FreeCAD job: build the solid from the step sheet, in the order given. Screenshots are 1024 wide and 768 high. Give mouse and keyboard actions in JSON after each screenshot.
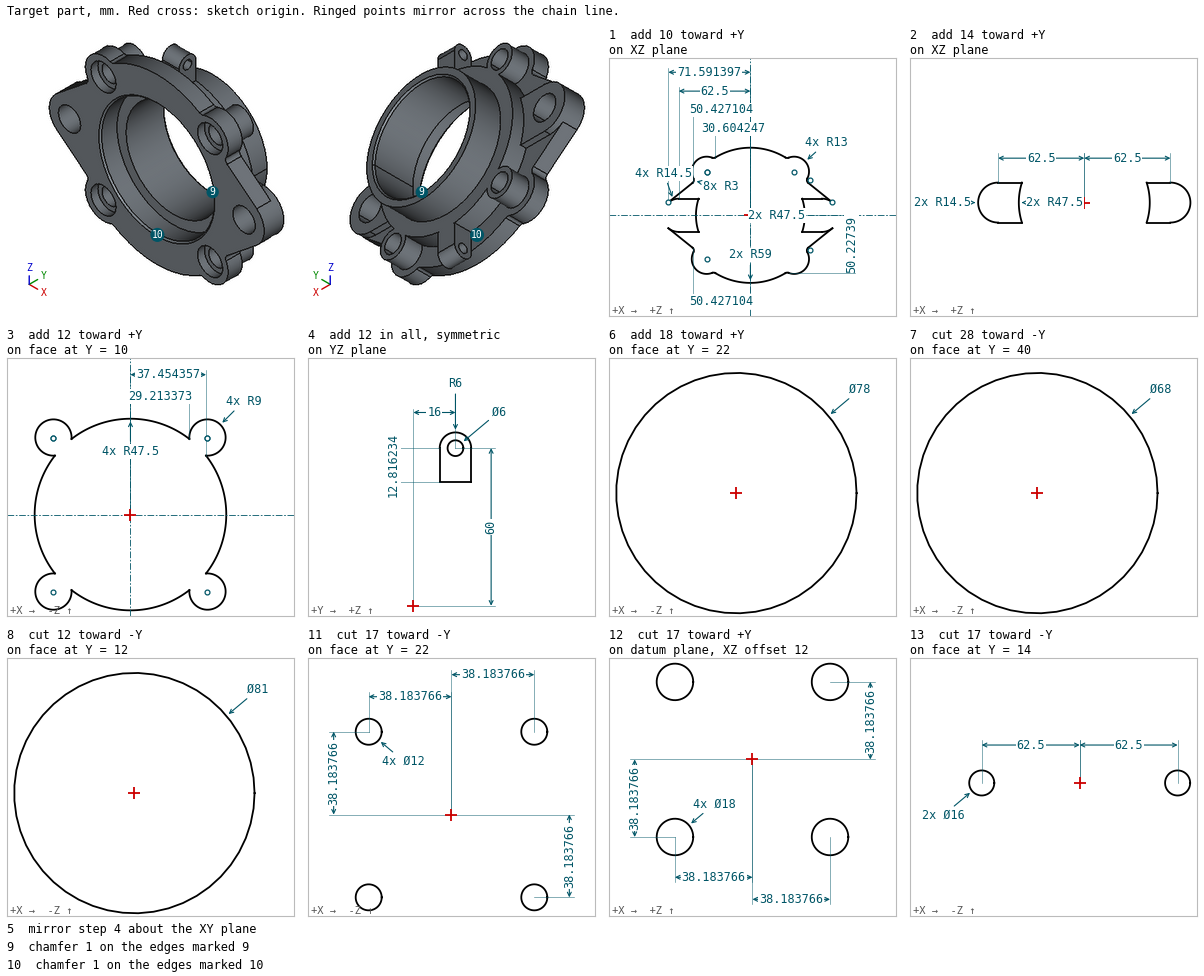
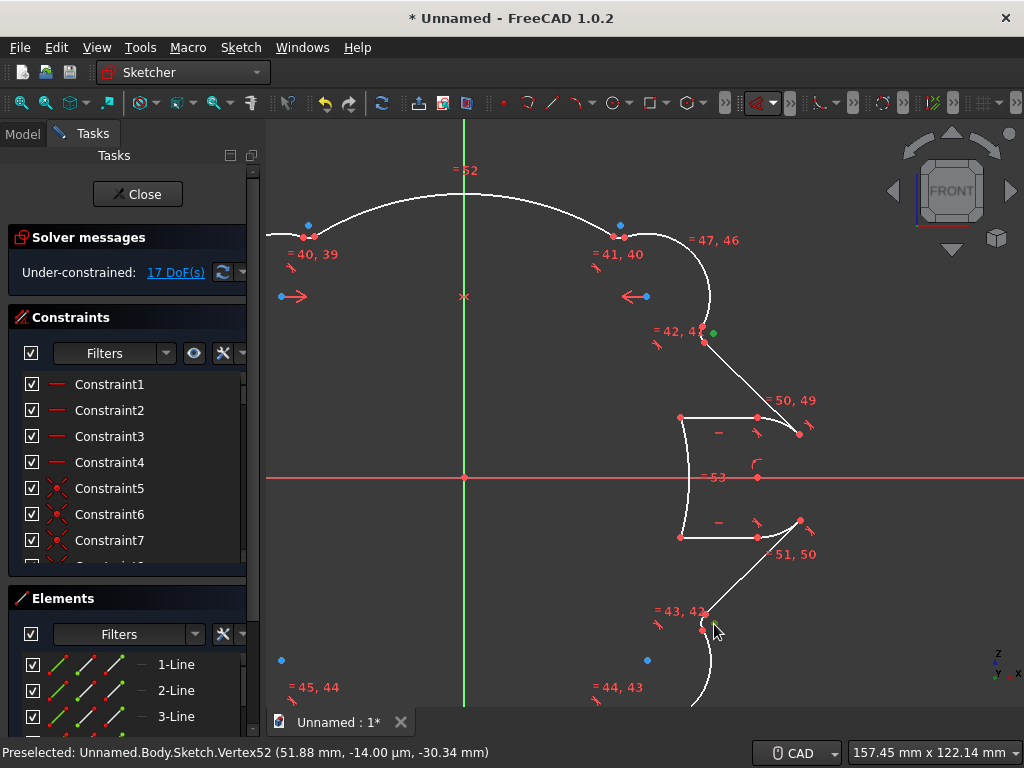
{"action": "left_click", "coordinate": [334, 478]}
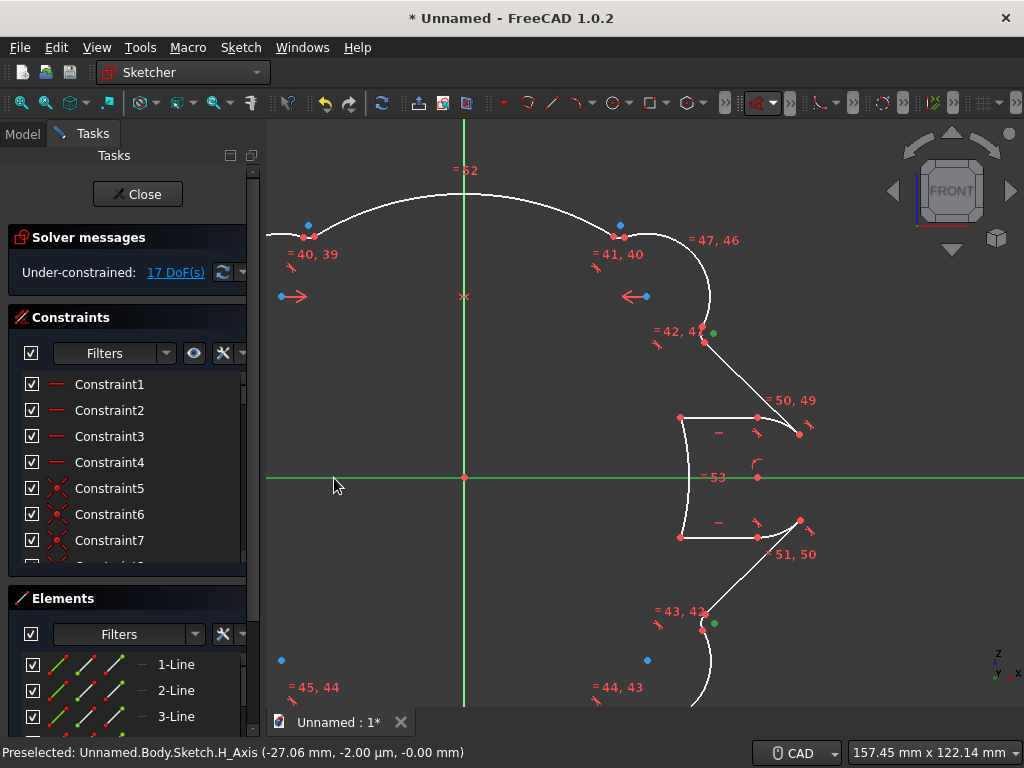
{"action": "key", "text": "s"}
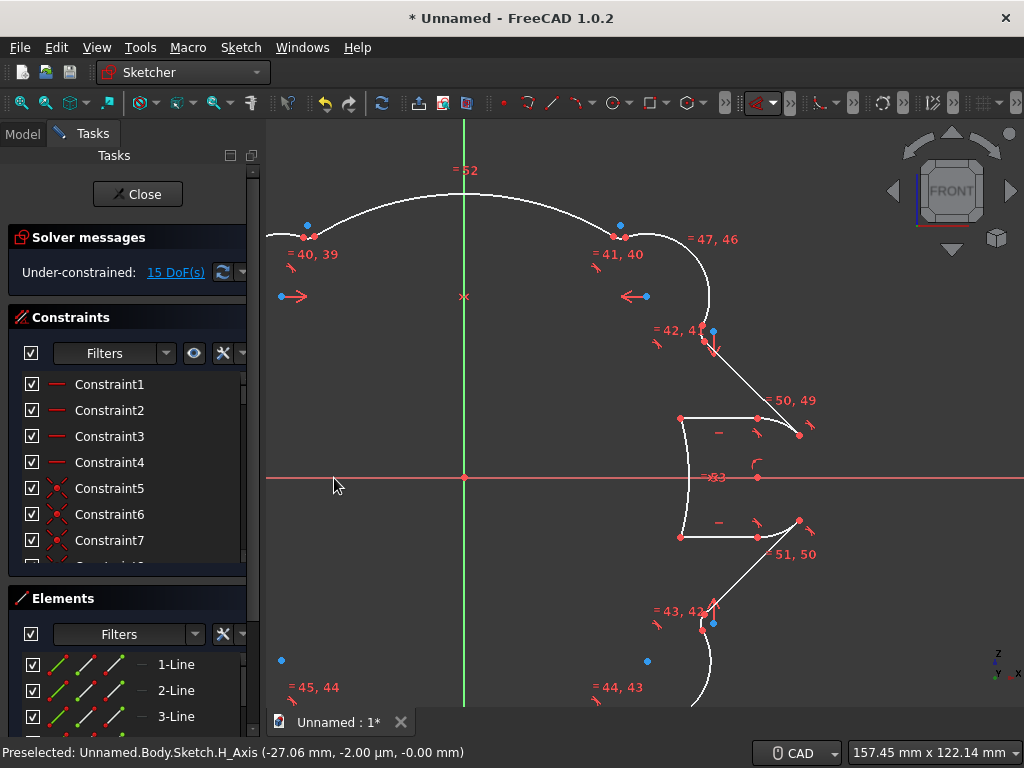
{"action": "scroll", "coordinate": [713, 334], "scroll_direction": "down", "scroll_amount": 3}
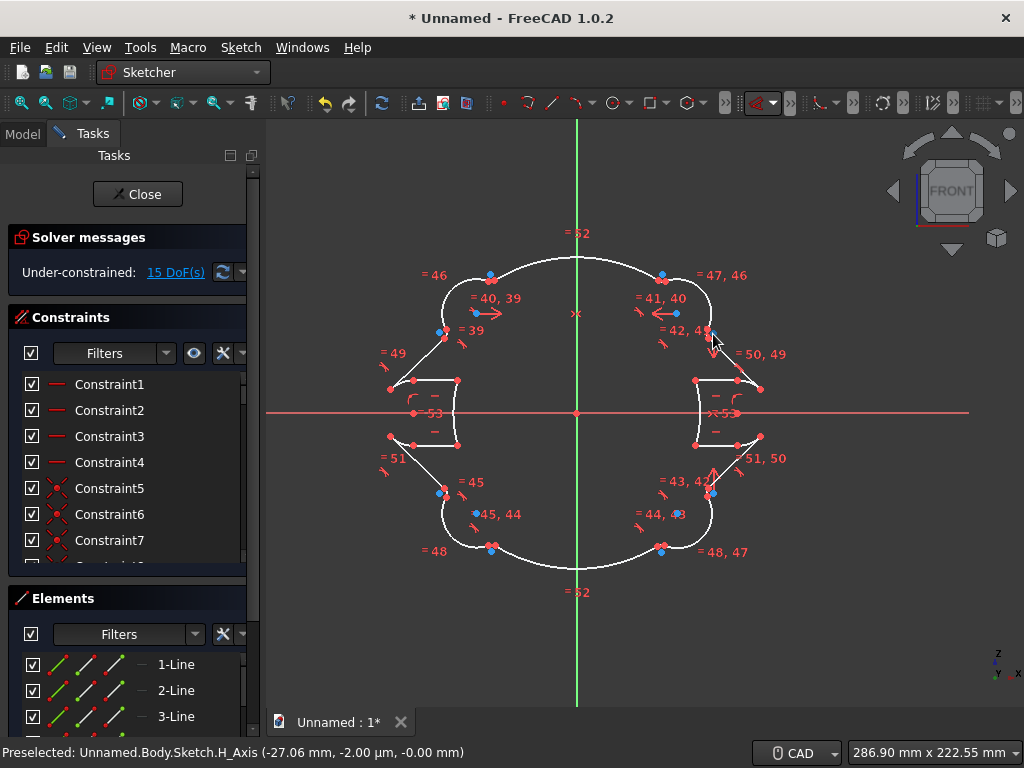
{"action": "left_click", "coordinate": [477, 314]}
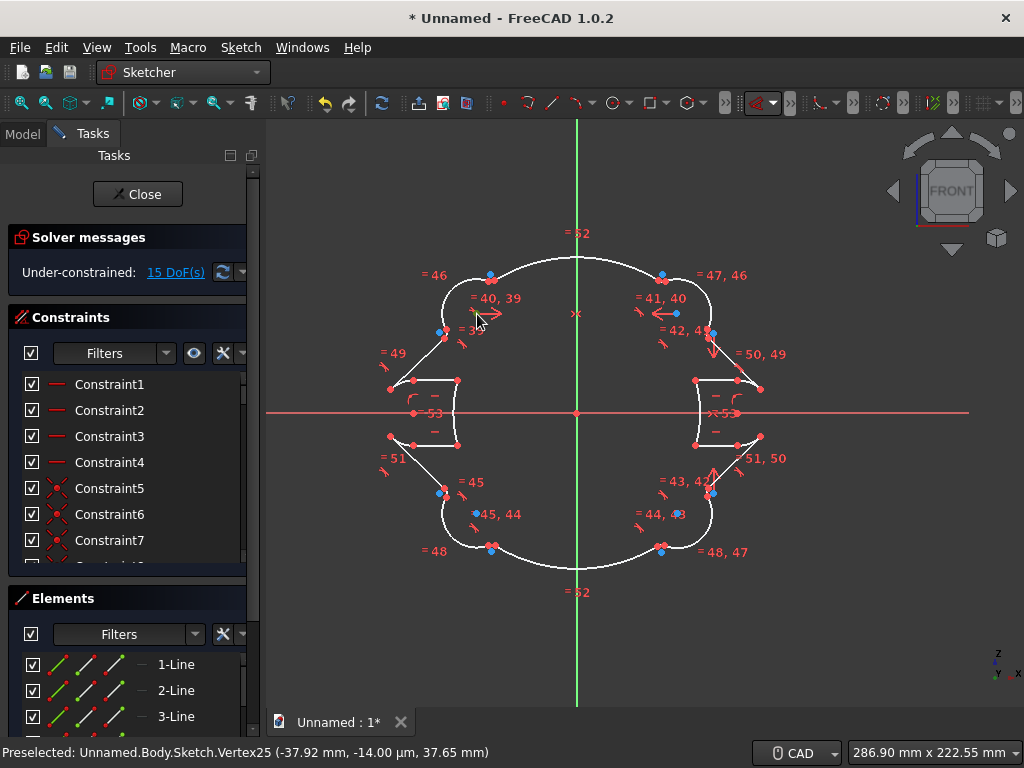
{"action": "left_click", "coordinate": [477, 513]}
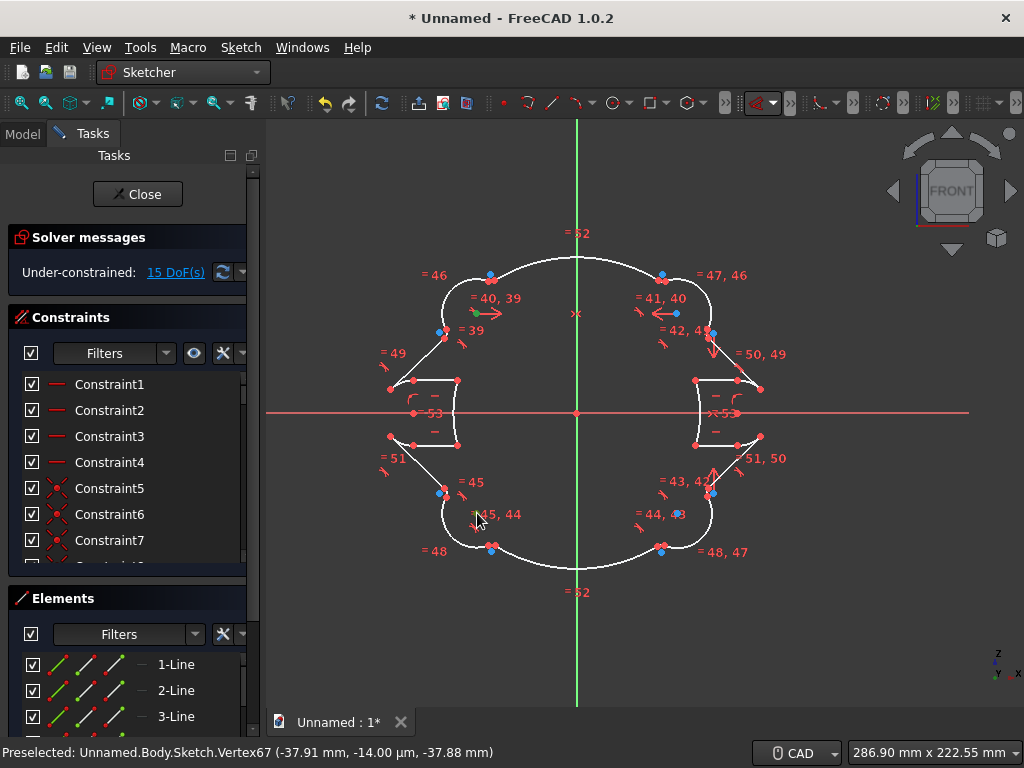
{"action": "left_click", "coordinate": [334, 413]}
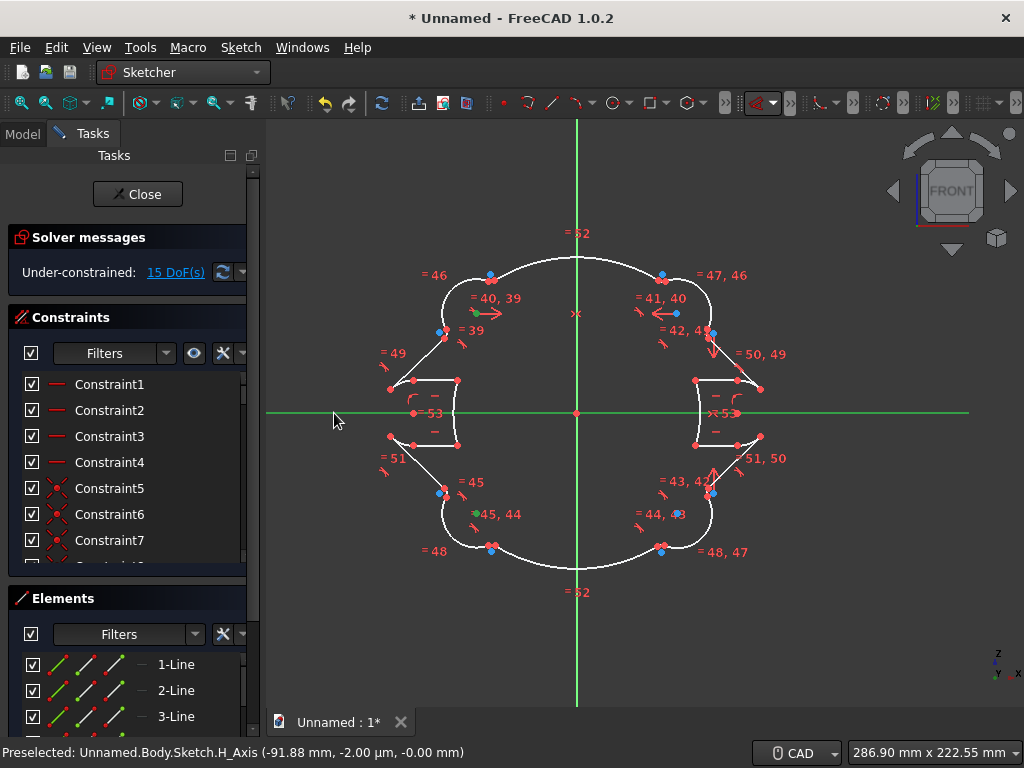
{"action": "key", "text": "s"}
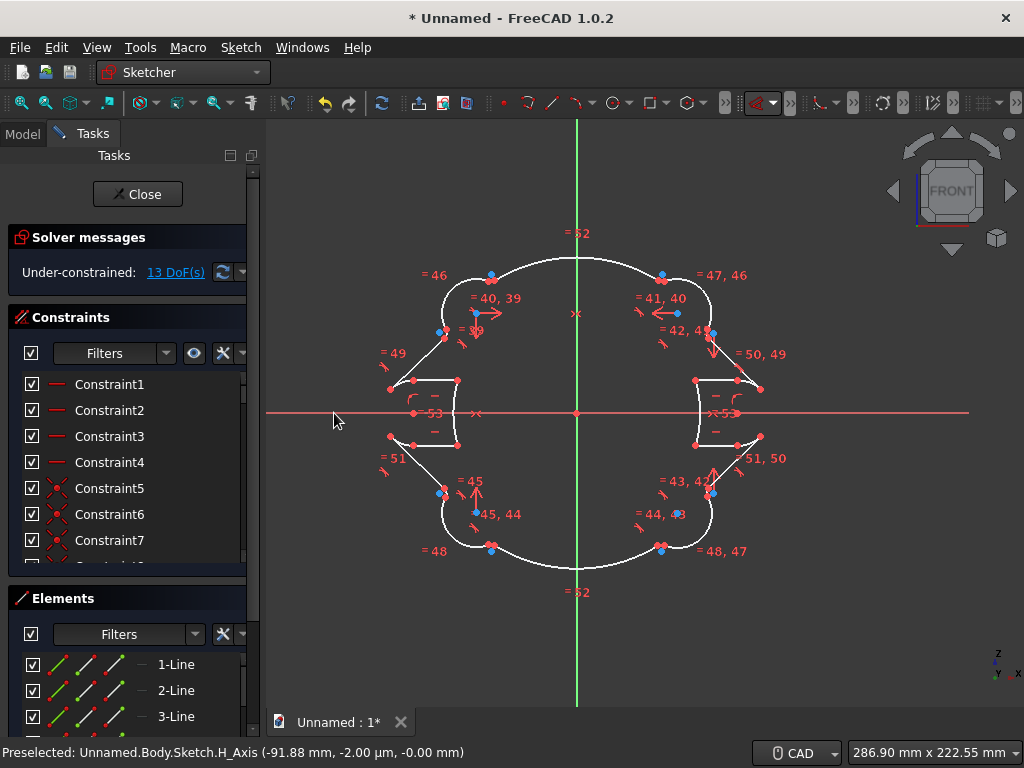
{"action": "left_click", "coordinate": [391, 389]}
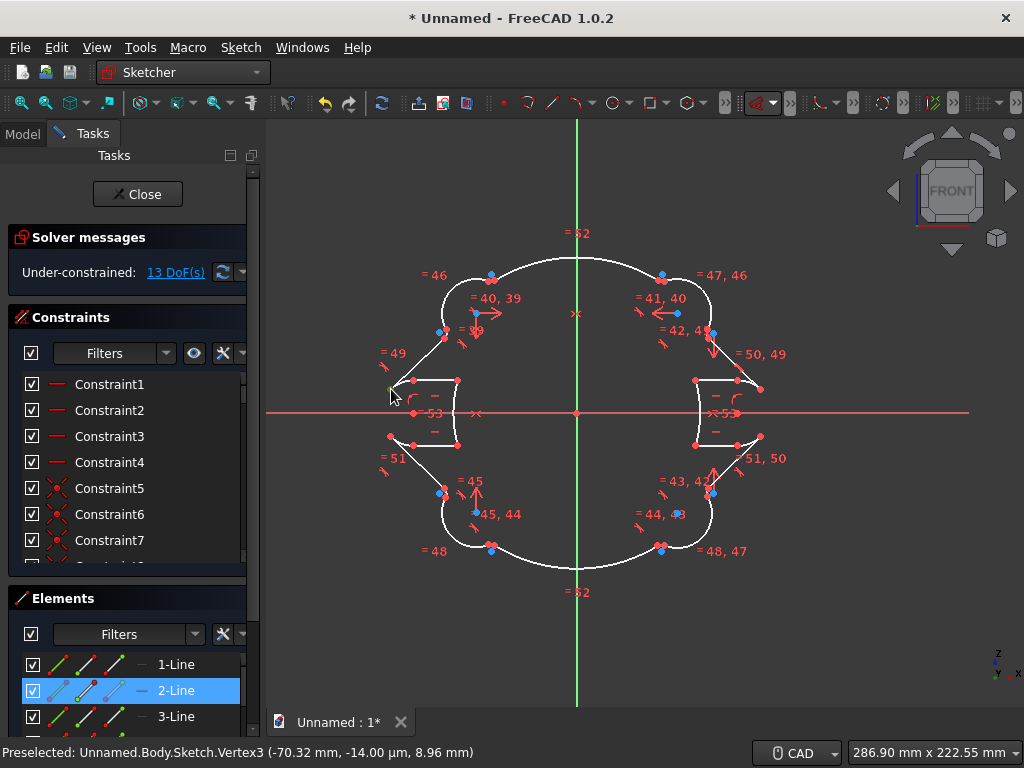
{"action": "left_click", "coordinate": [761, 390]}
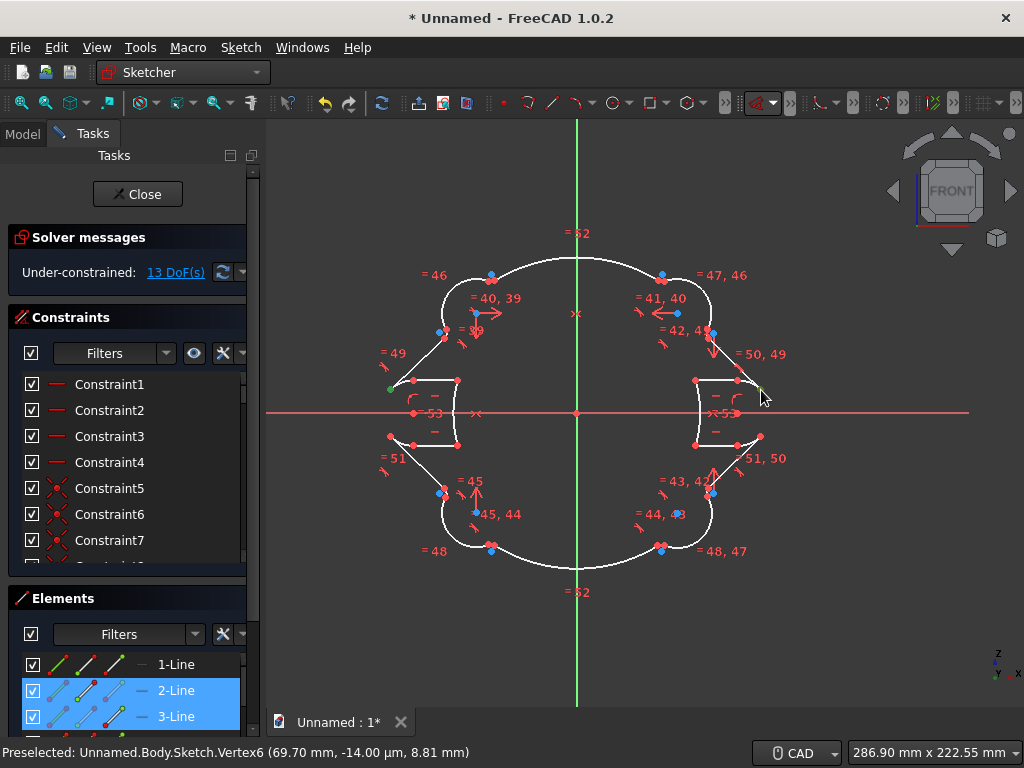
{"action": "left_click", "coordinate": [577, 641]}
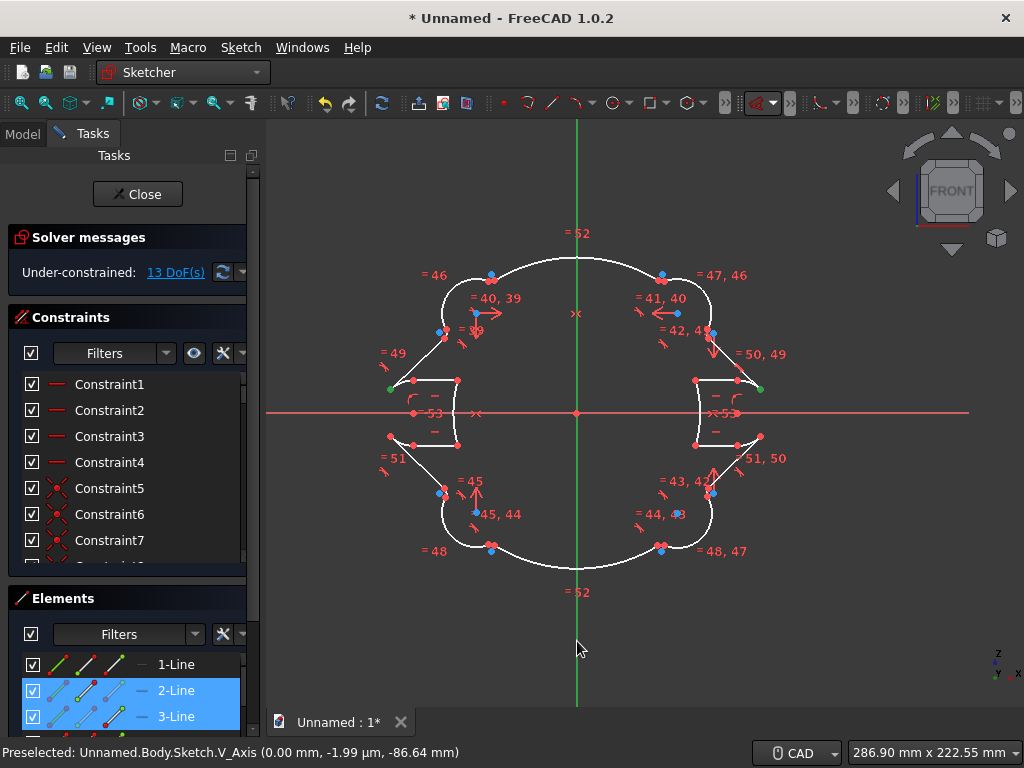
{"action": "key", "text": "s"}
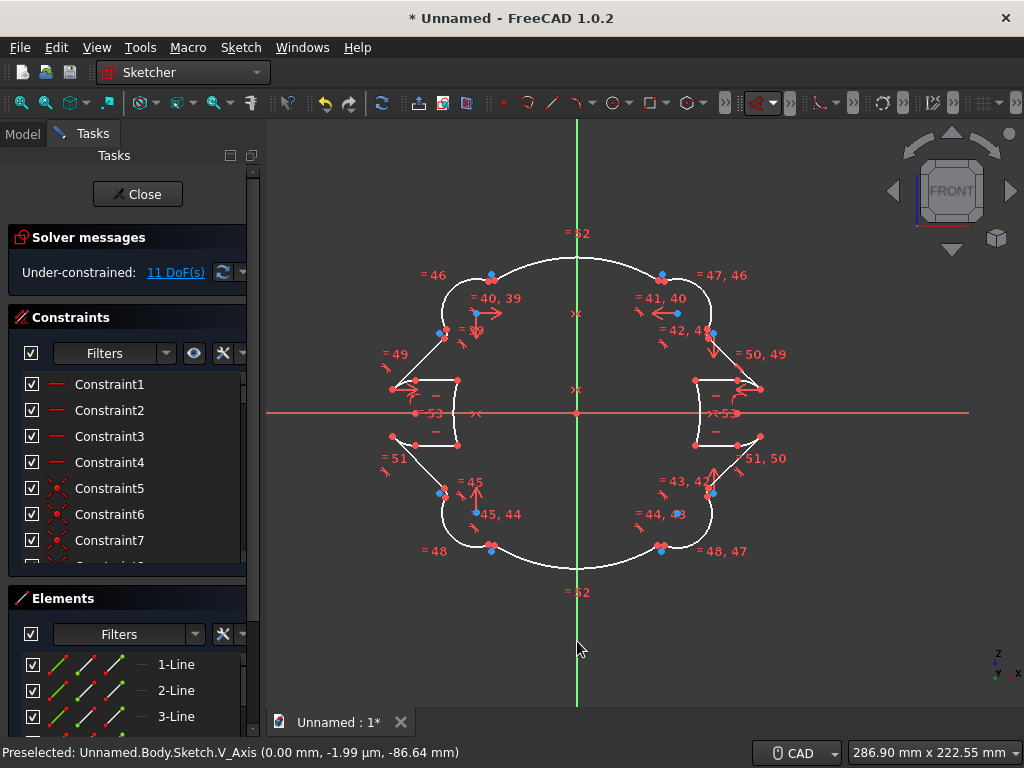
{"action": "key", "text": "d"}